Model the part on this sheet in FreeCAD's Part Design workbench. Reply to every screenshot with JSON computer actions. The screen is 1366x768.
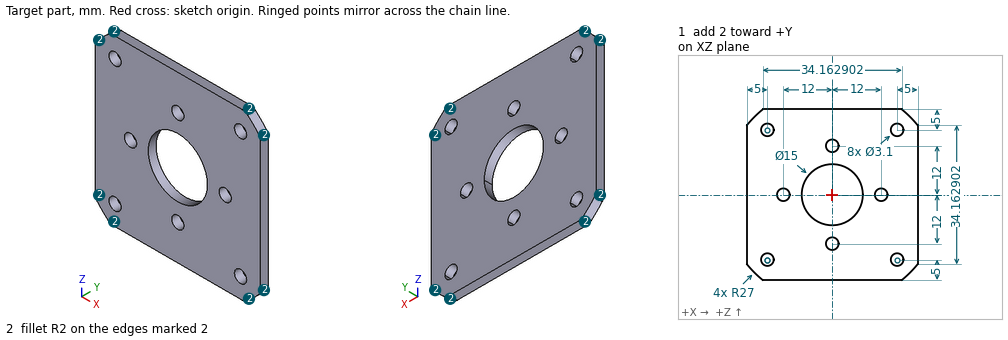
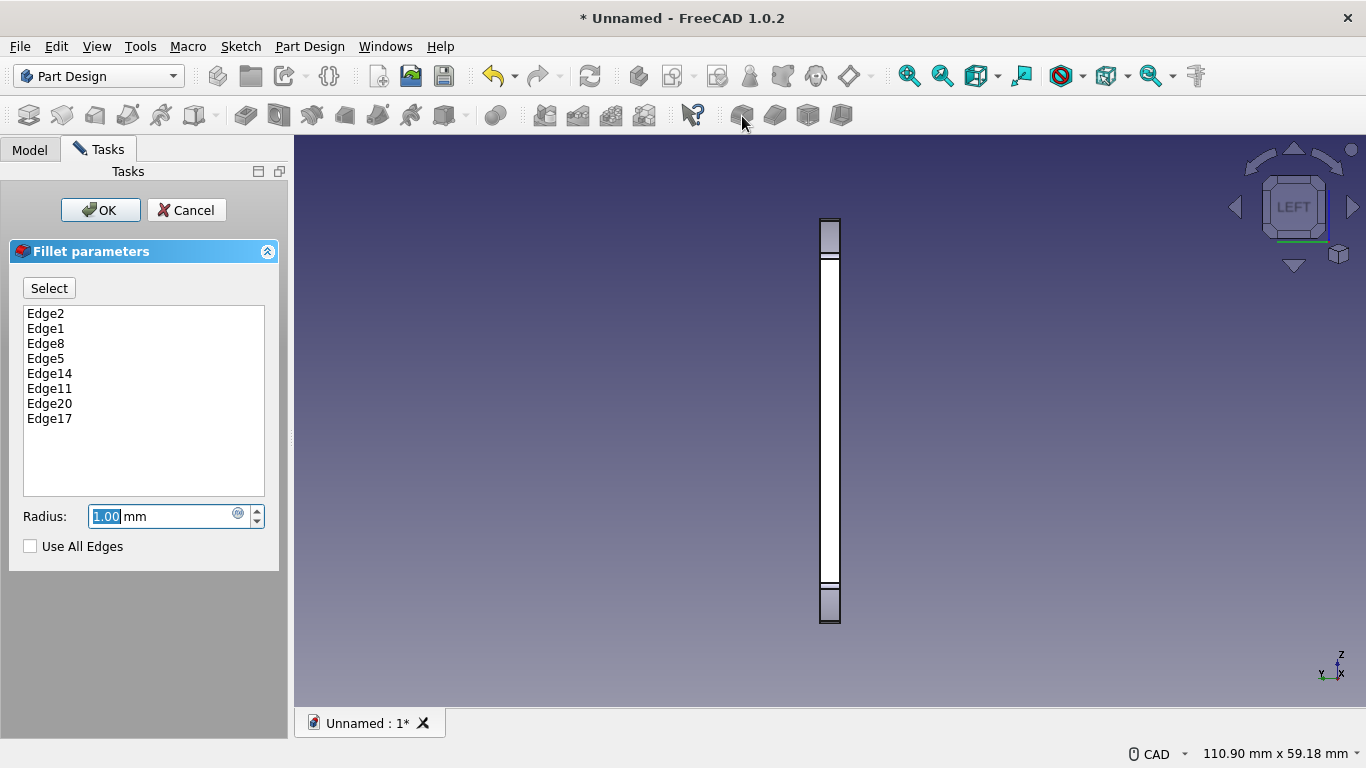
{"action": "type", "text": "2"}
{"action": "key", "text": "Tab"}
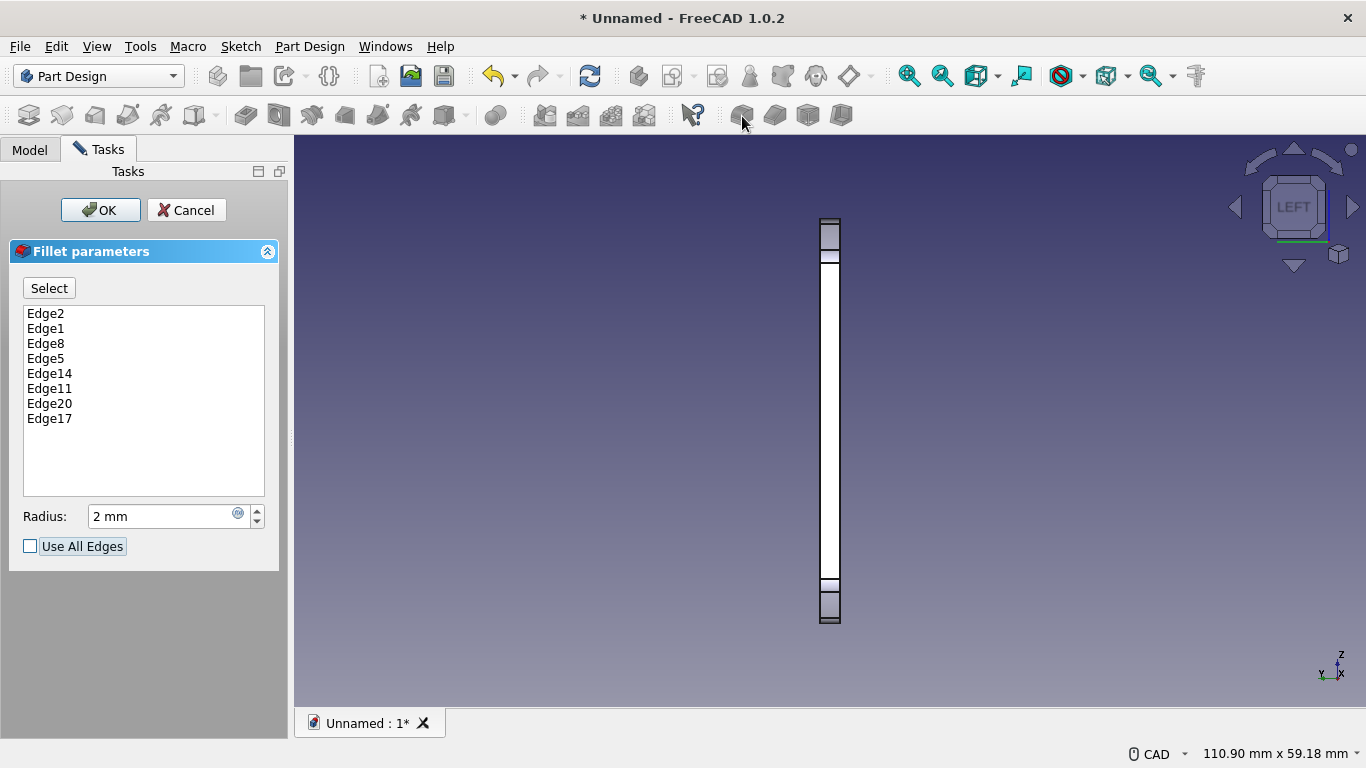
{"action": "left_click", "coordinate": [101, 210]}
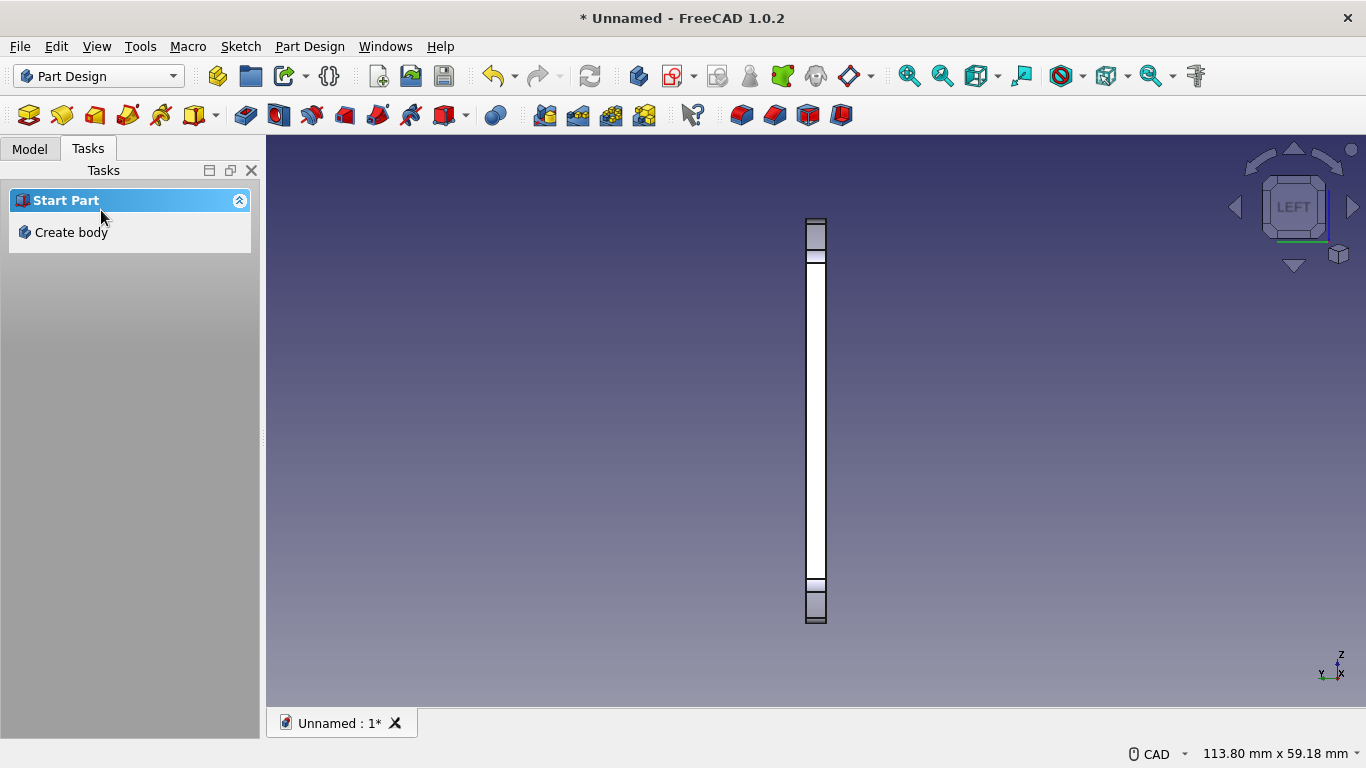
{"action": "key", "text": "0"}